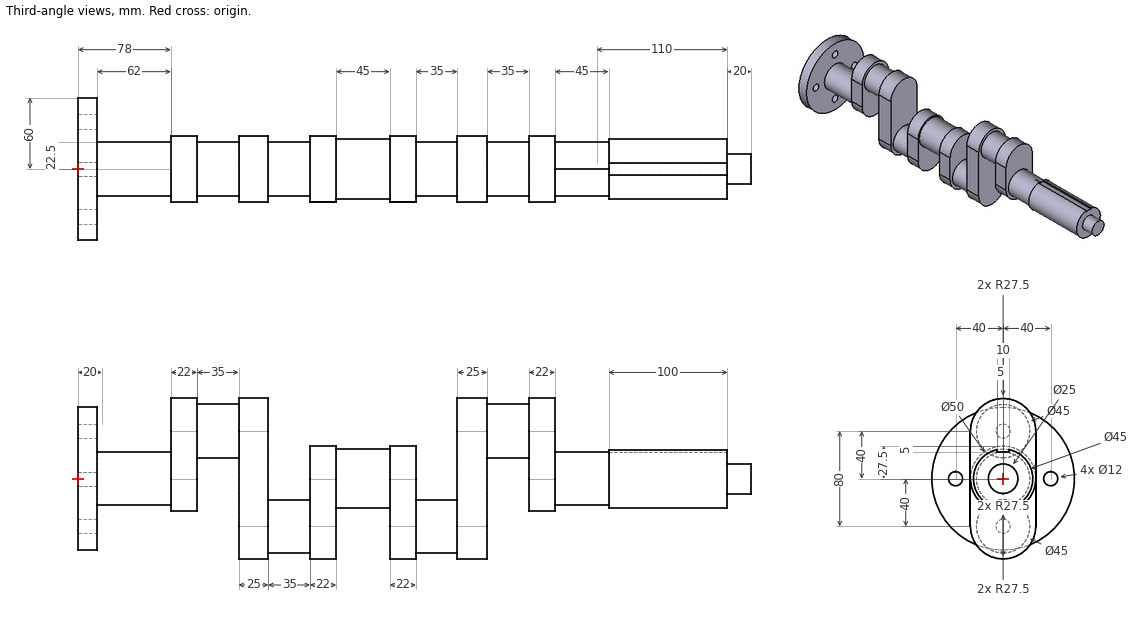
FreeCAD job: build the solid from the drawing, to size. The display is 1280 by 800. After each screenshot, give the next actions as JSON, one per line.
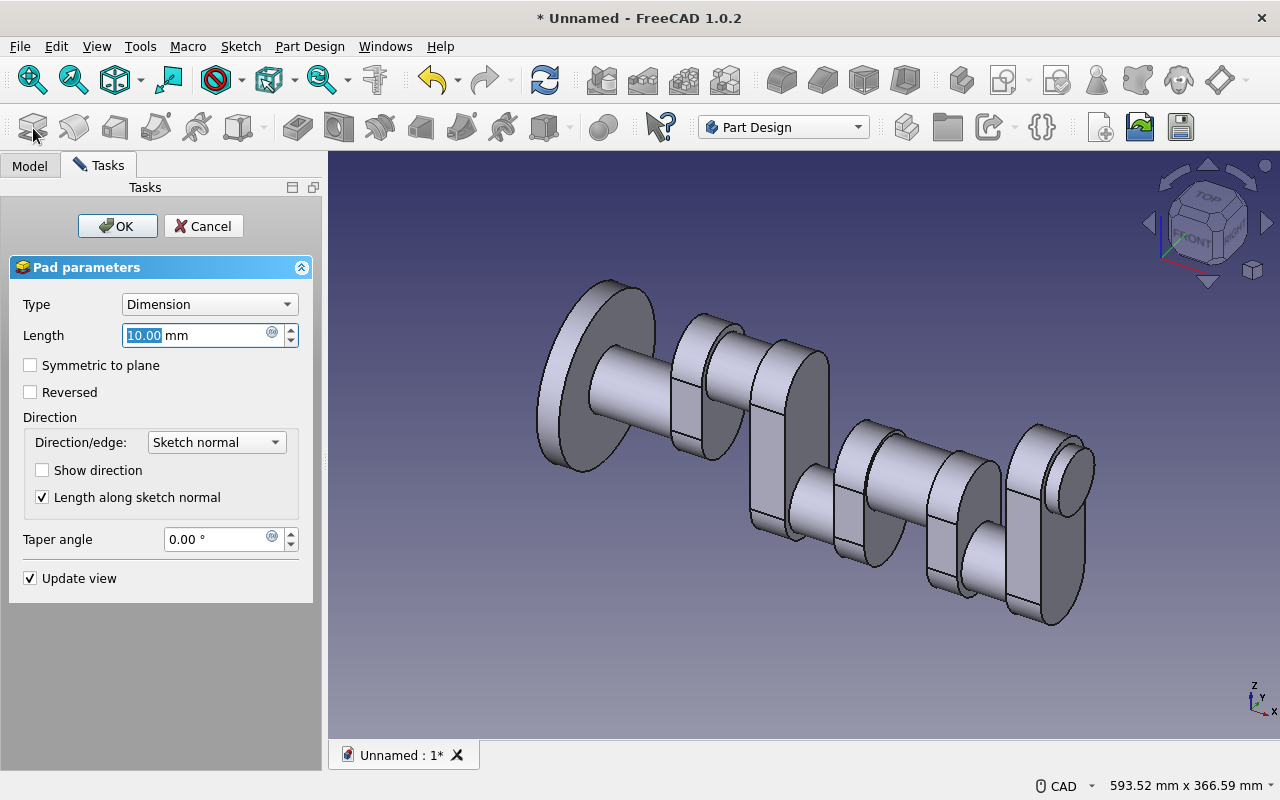
{"action": "type", "text": "35"}
{"action": "key", "text": "Tab"}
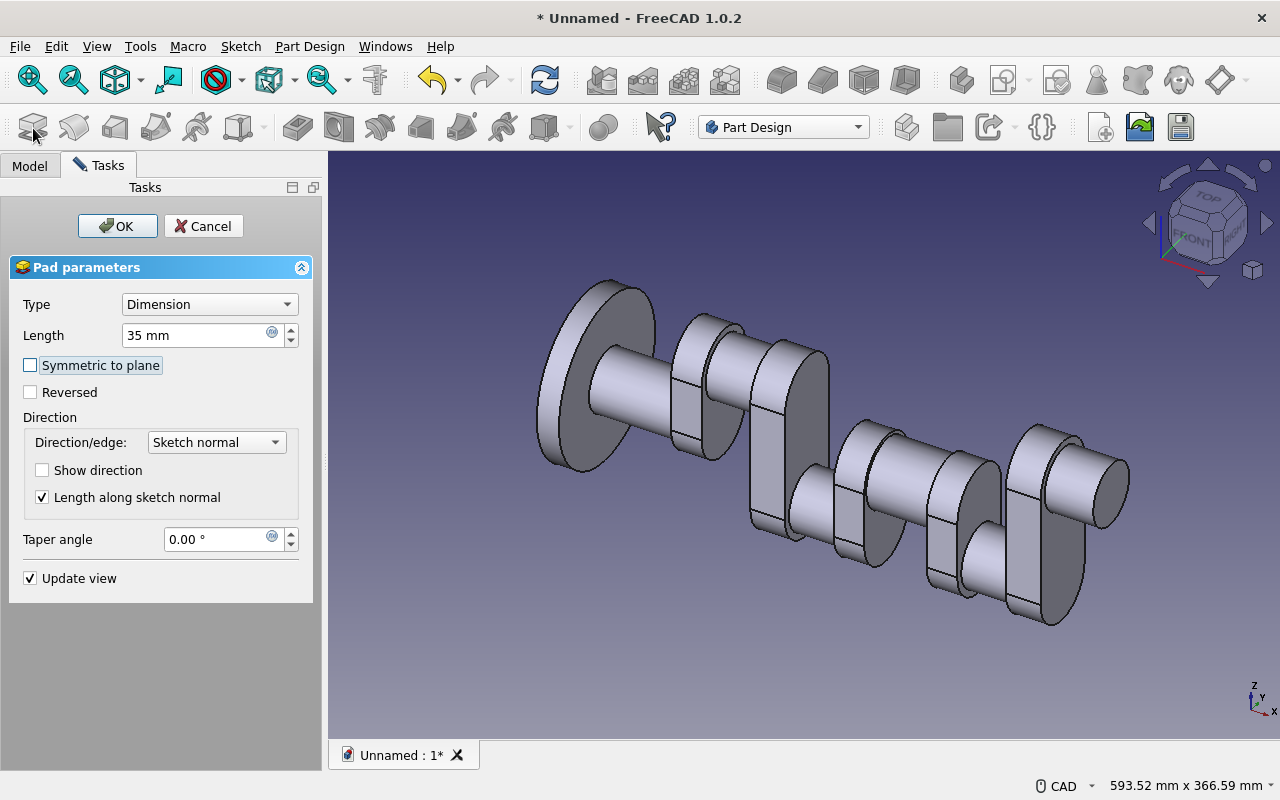
{"action": "left_click", "coordinate": [118, 226]}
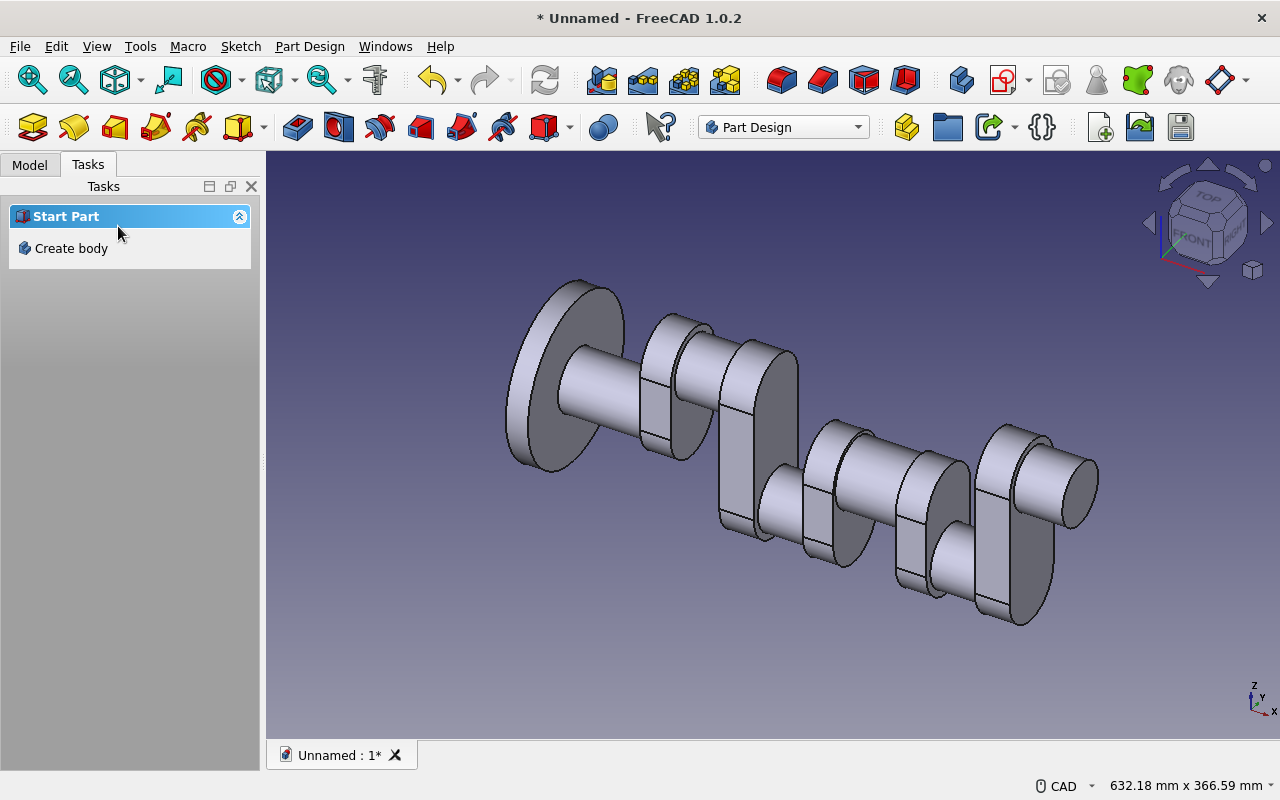
{"action": "left_click", "coordinate": [1080, 493]}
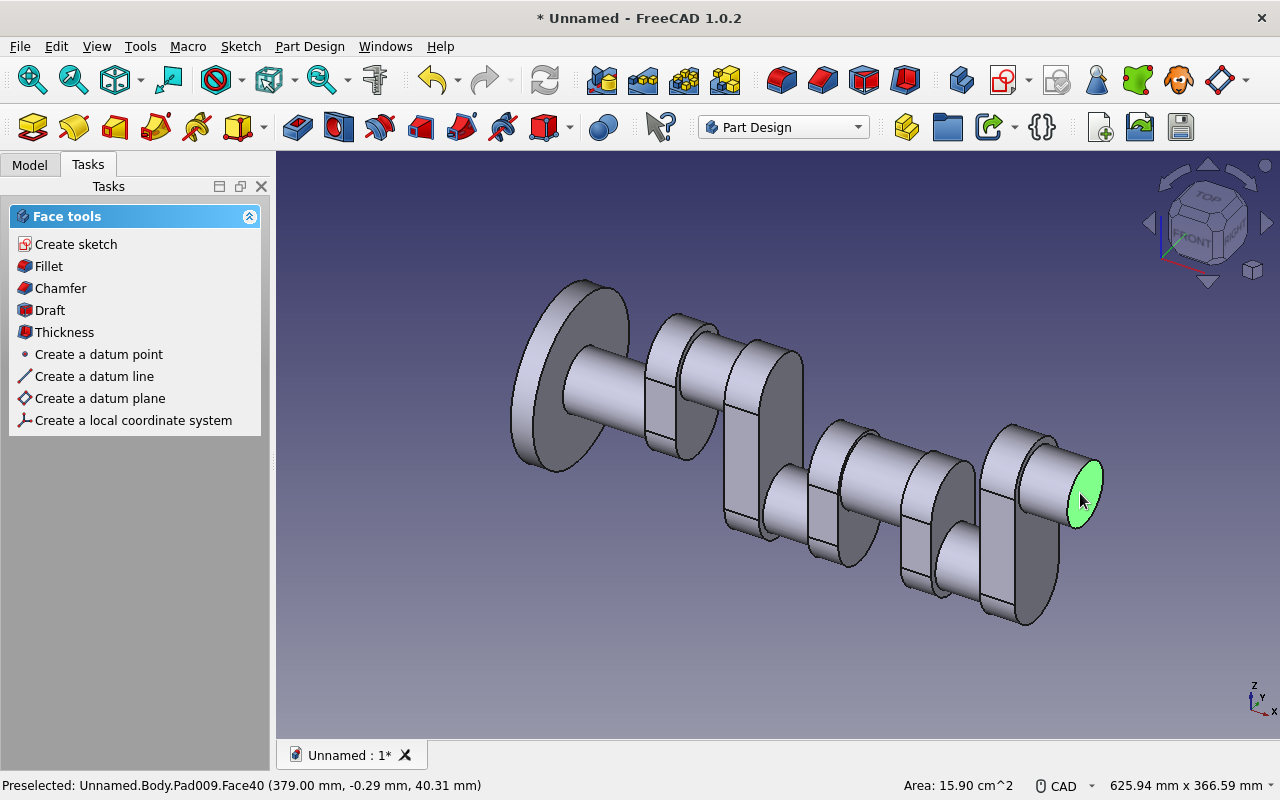
{"action": "left_click", "coordinate": [1002, 80]}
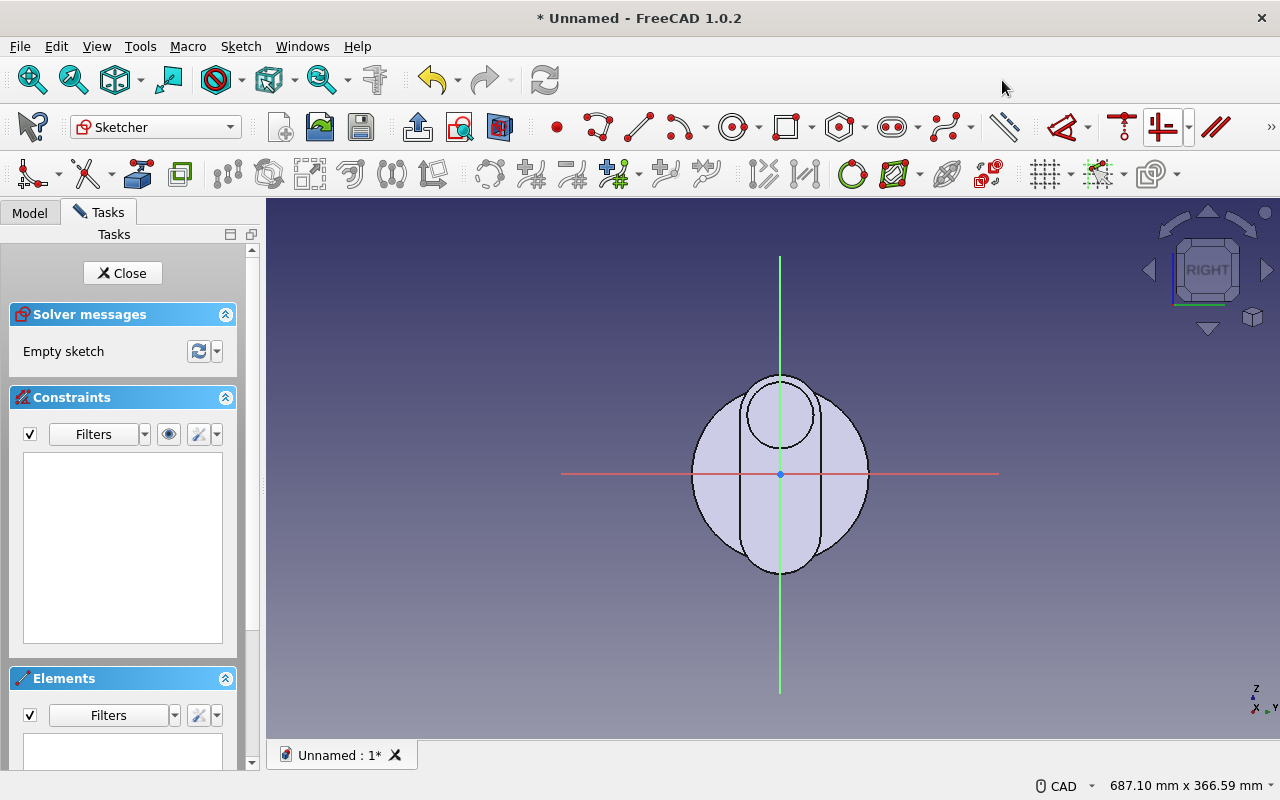
{"action": "scroll", "coordinate": [842, 426], "scroll_direction": "up", "scroll_amount": 4}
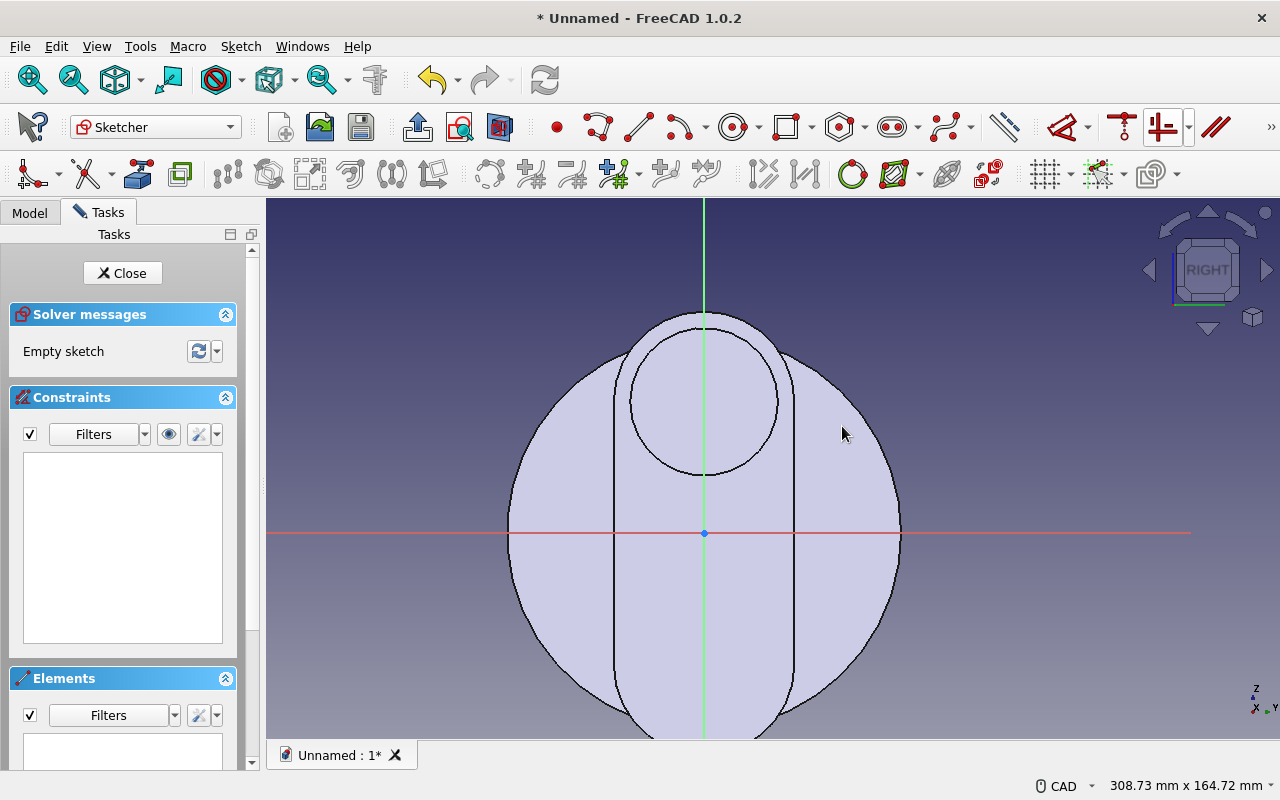
{"action": "left_click", "coordinate": [892, 128]}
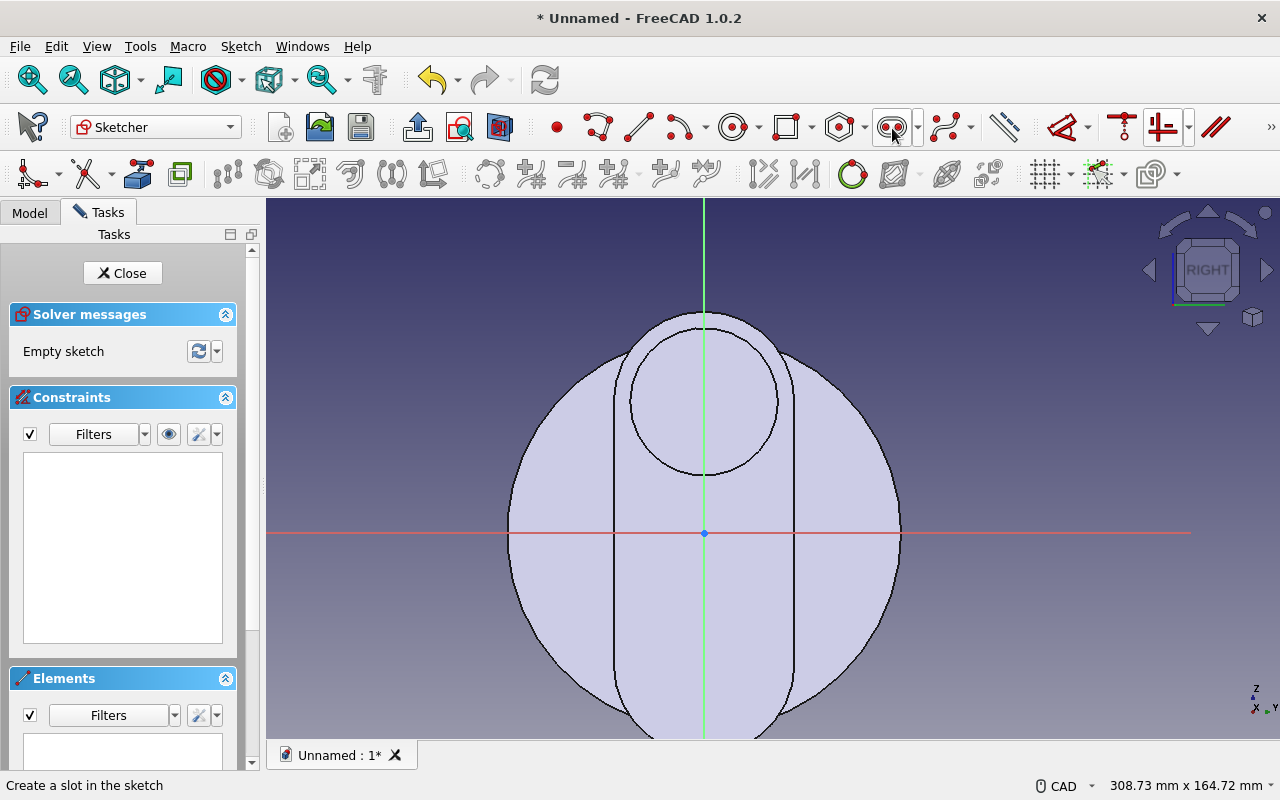
{"action": "left_click", "coordinate": [704, 533]}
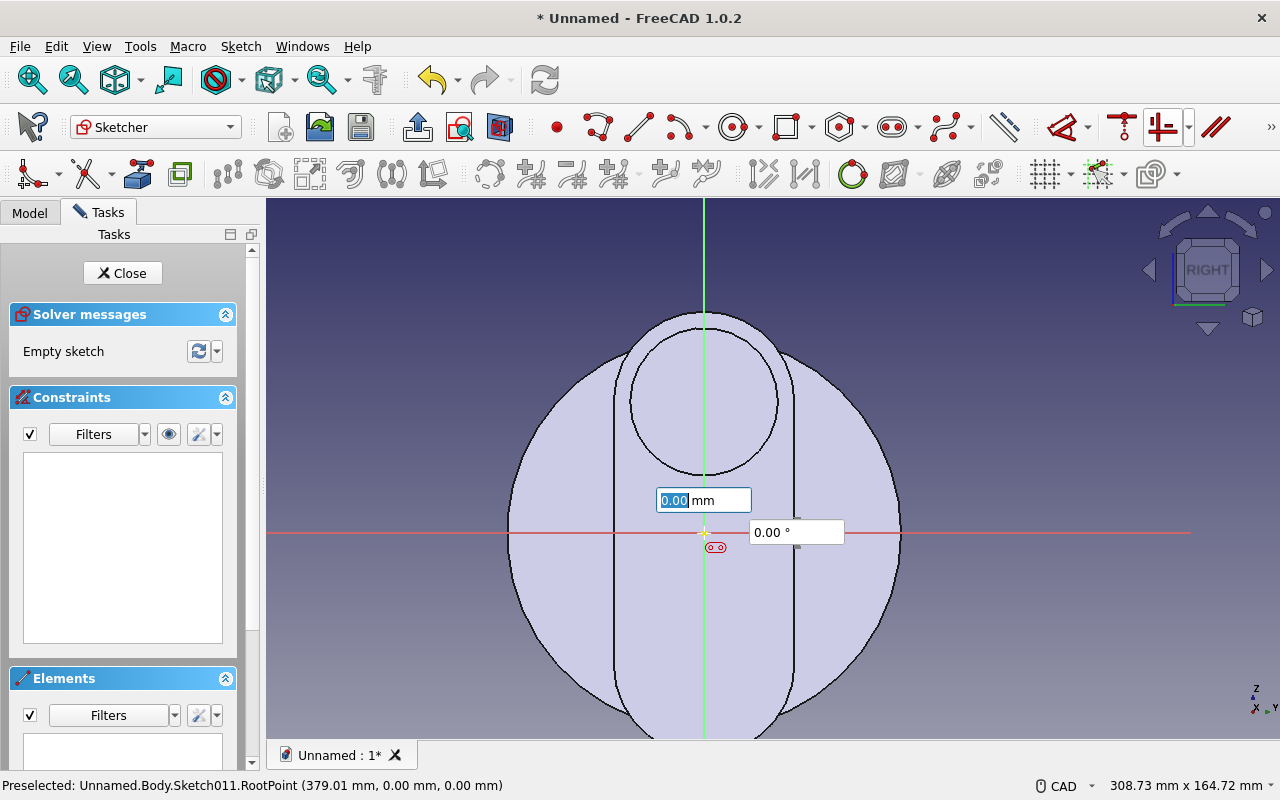
{"action": "left_click", "coordinate": [713, 402]}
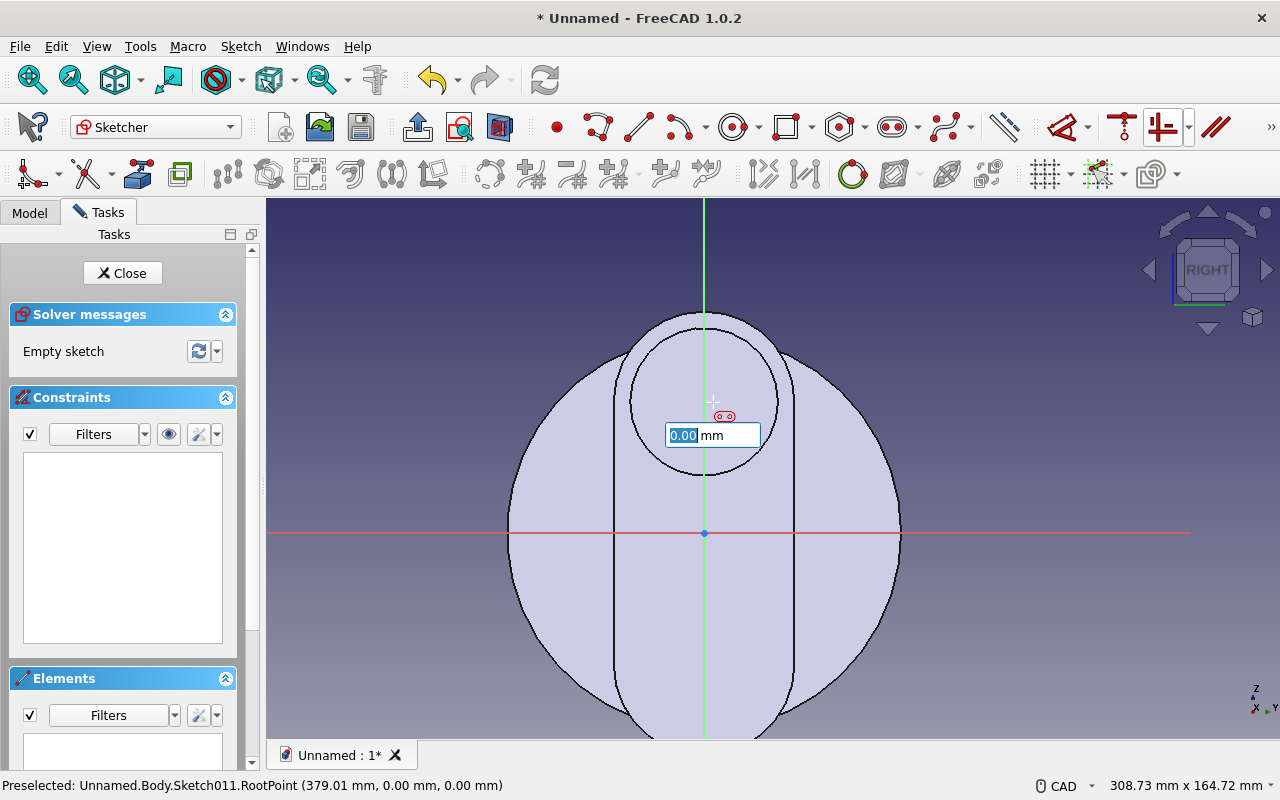
{"action": "left_click", "coordinate": [794, 468]}
{"action": "key", "text": "Escape"}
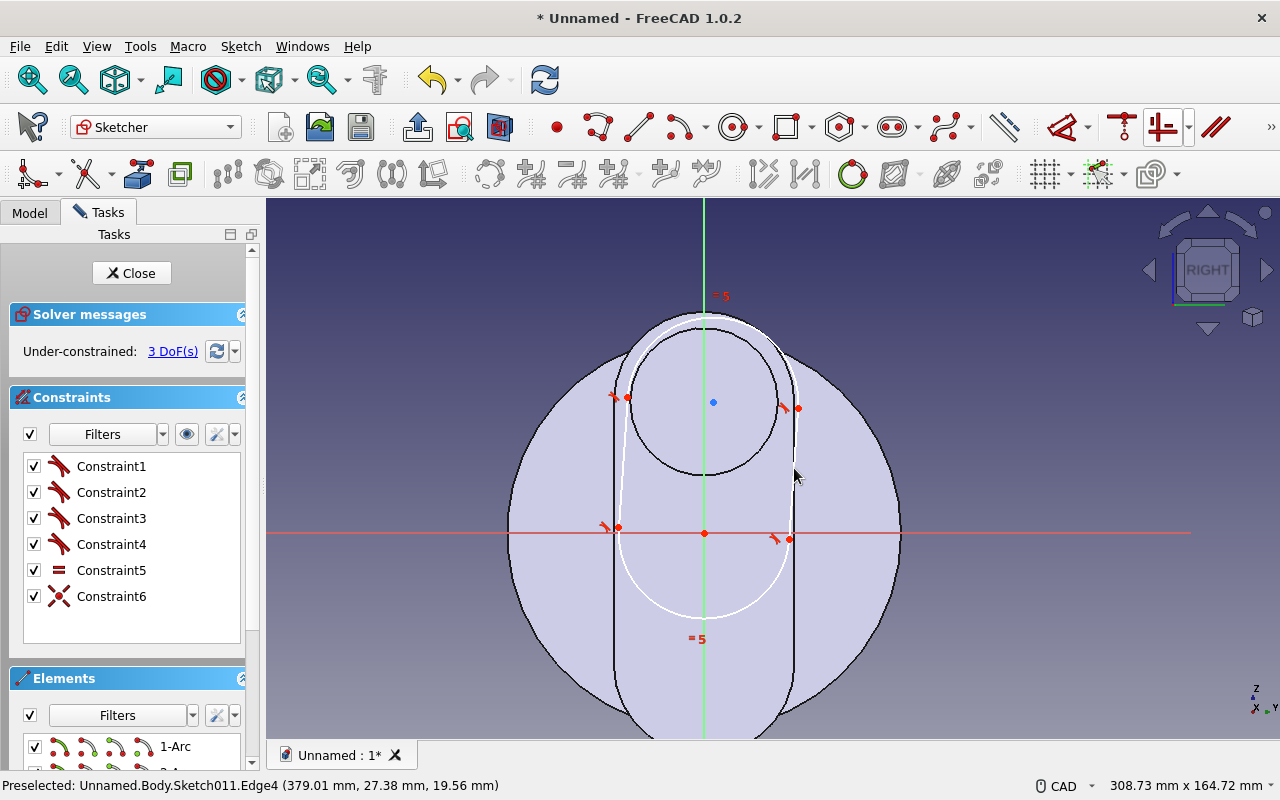
{"action": "left_click", "coordinate": [622, 488]}